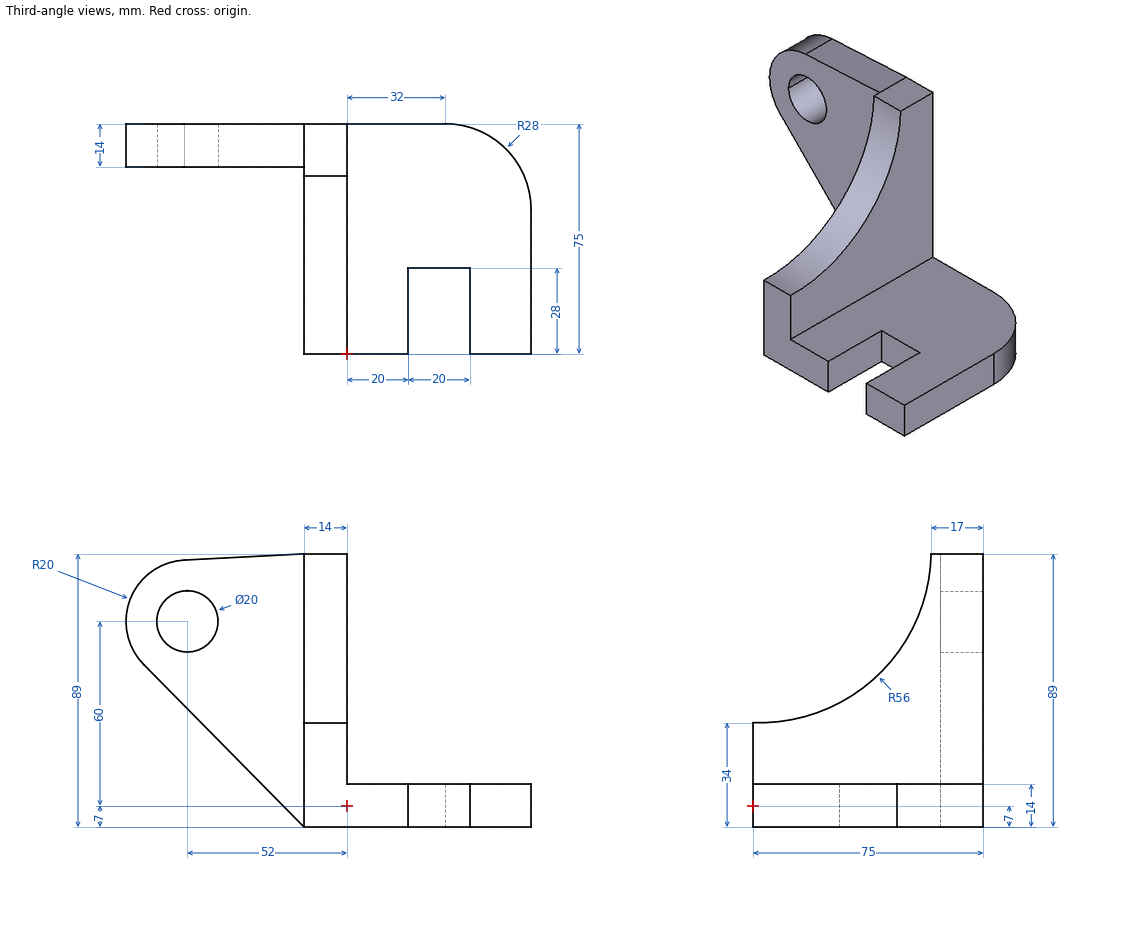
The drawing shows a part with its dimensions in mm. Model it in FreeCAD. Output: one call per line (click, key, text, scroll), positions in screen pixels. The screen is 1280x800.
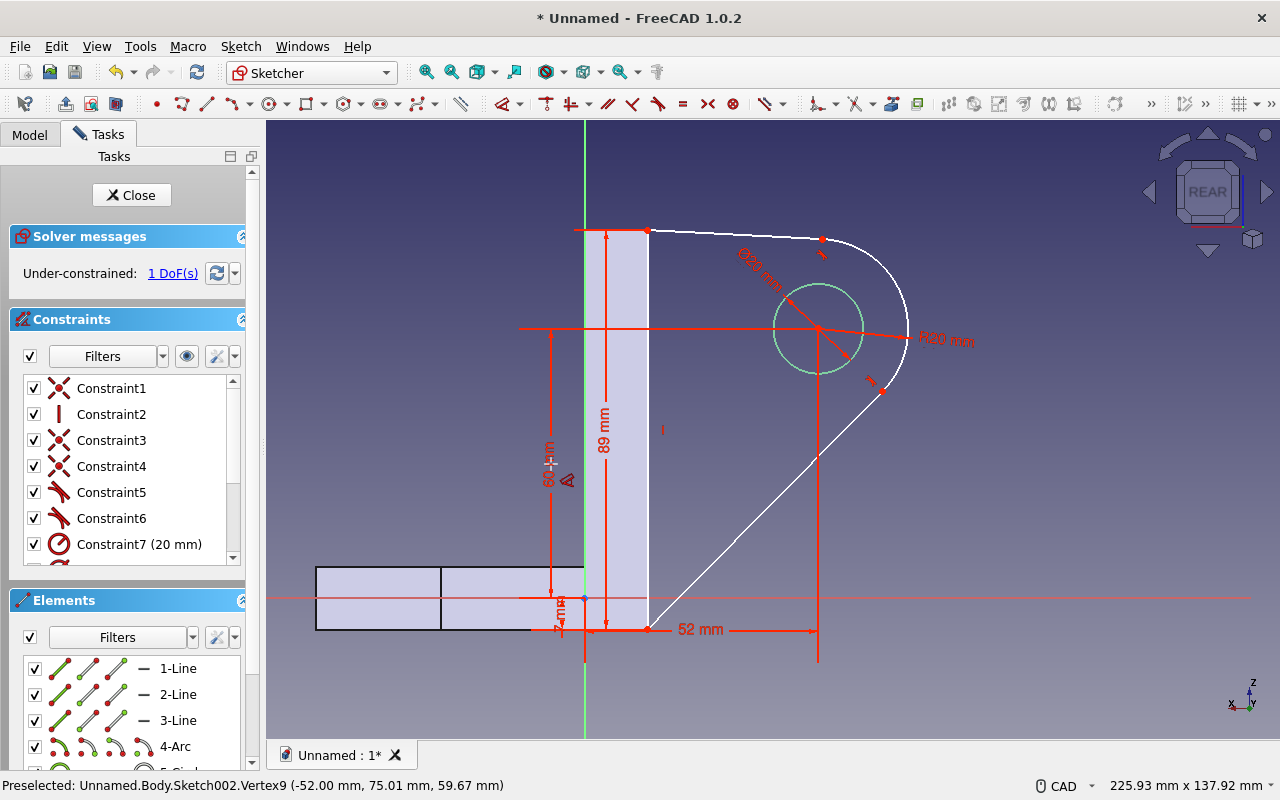
click(648, 230)
click(616, 196)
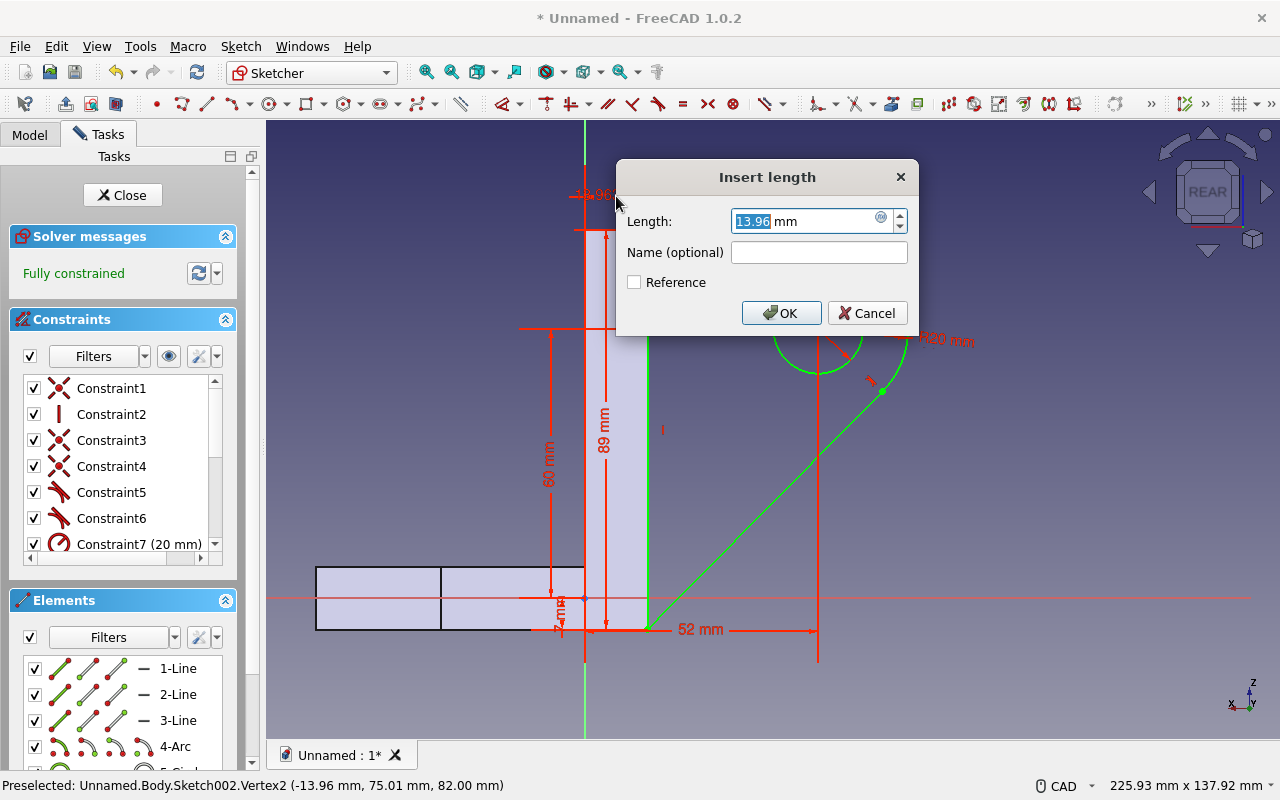
text(14)
key(Return)
key(Escape)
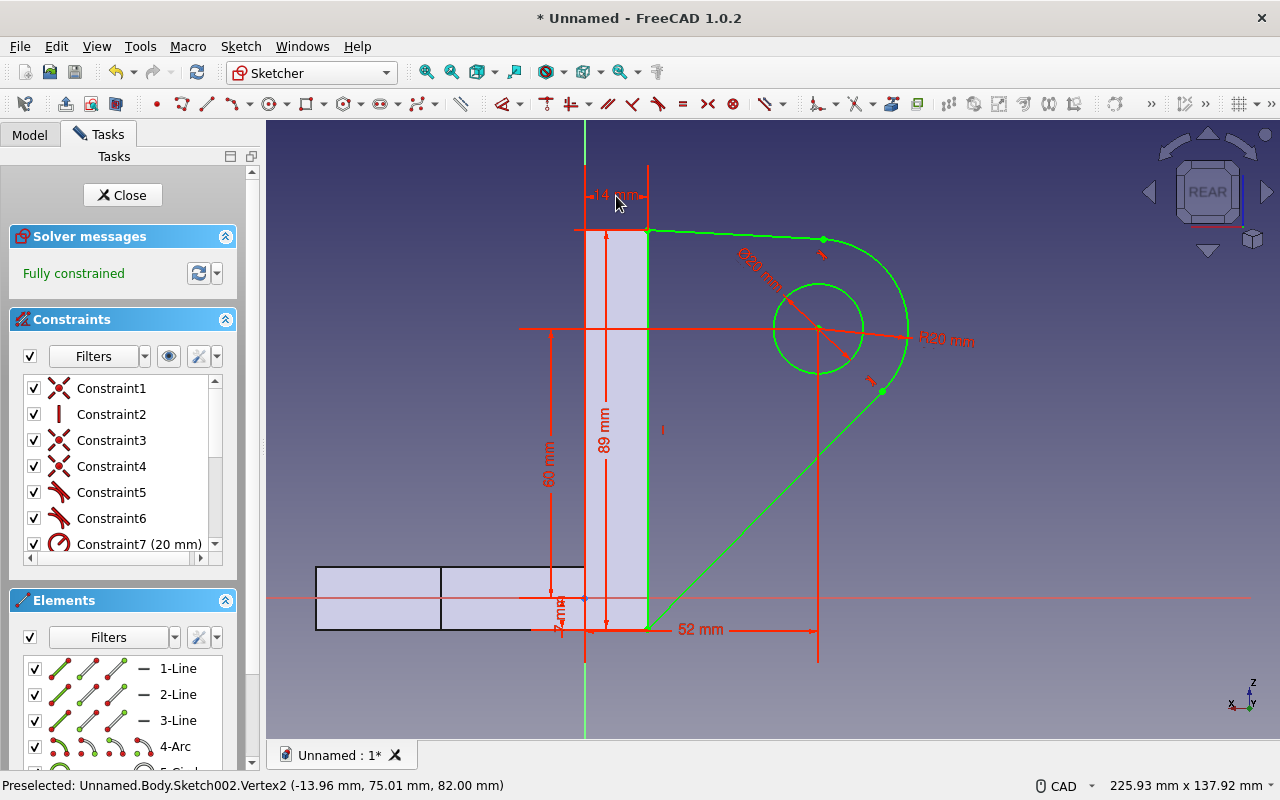
click(123, 195)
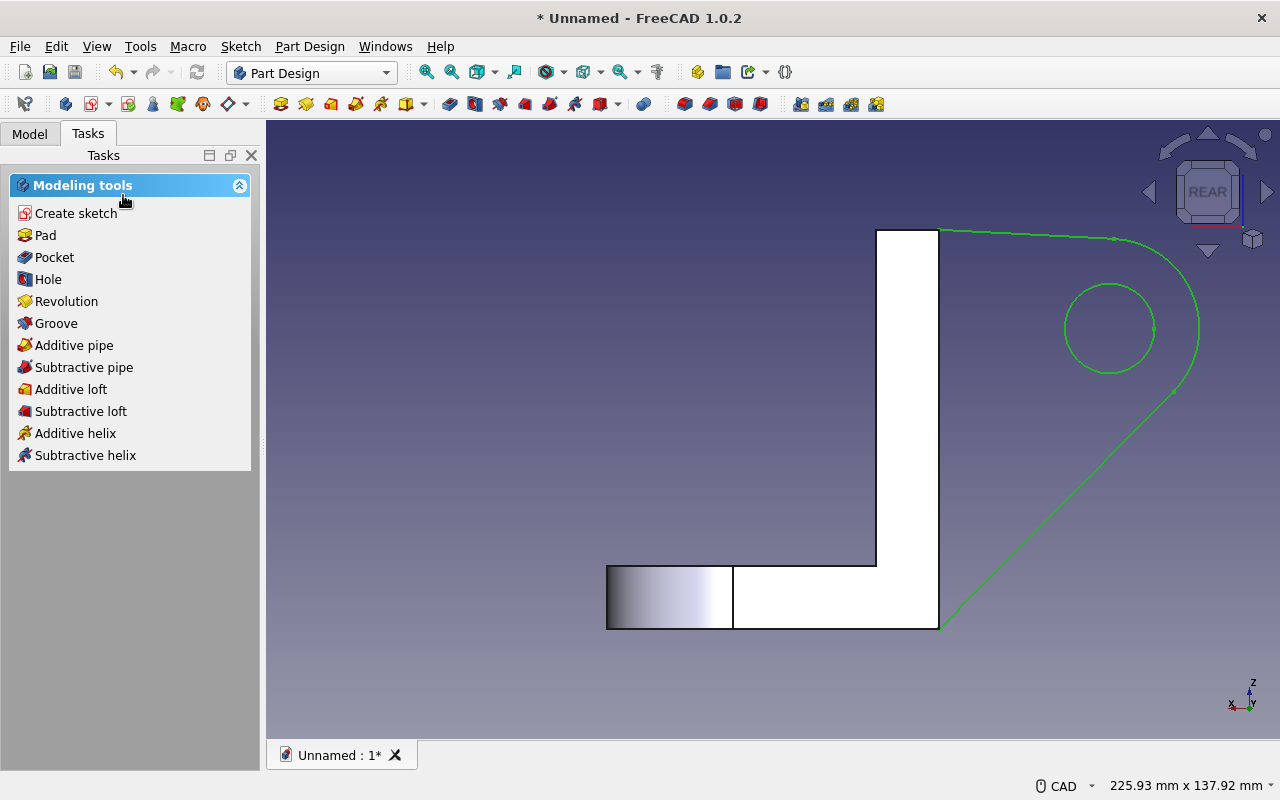
click(281, 104)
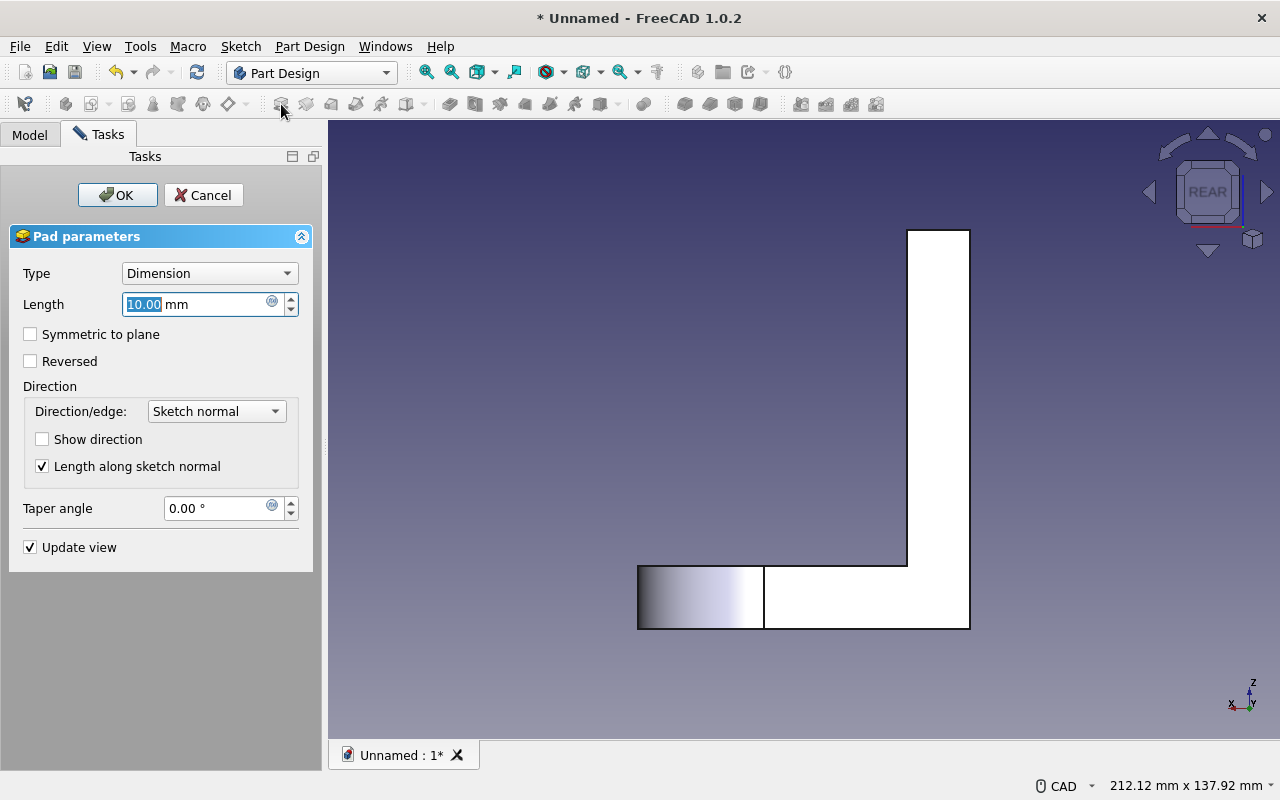
text(14)
key(Tab)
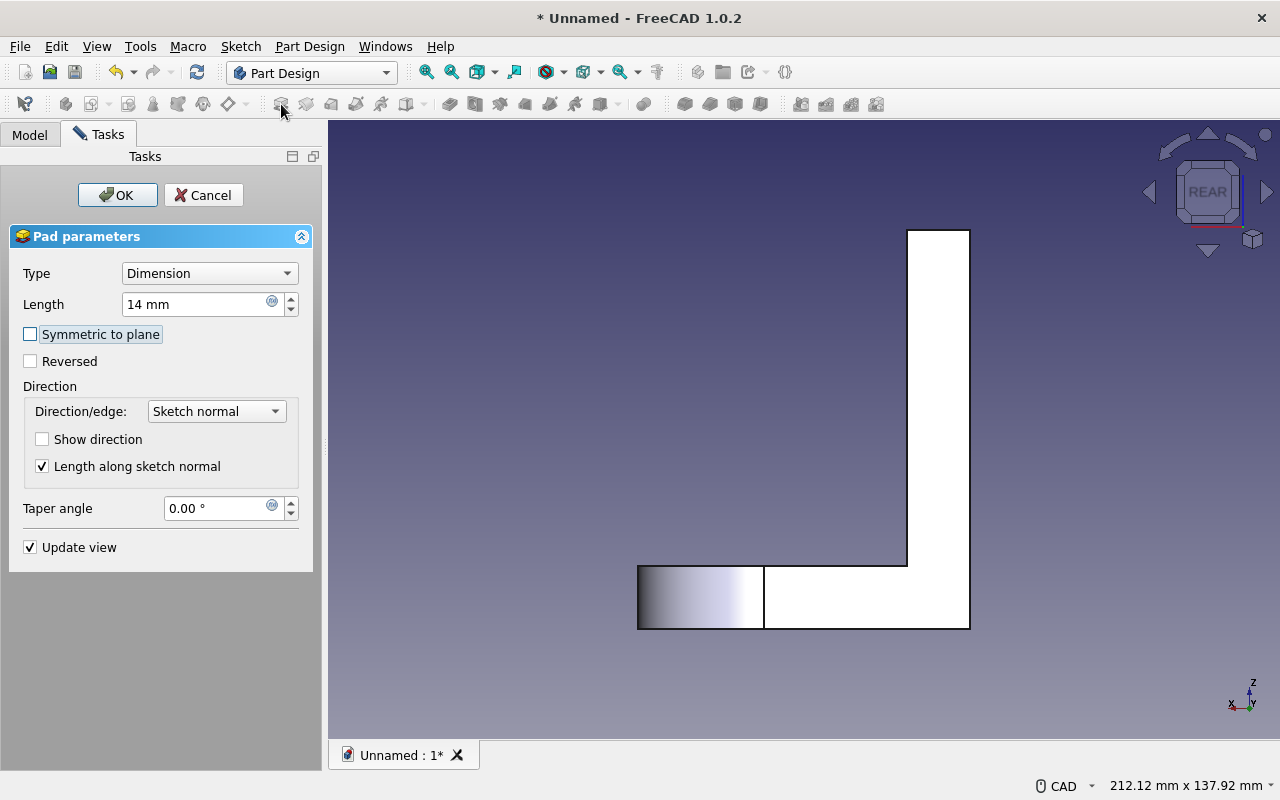
click(31, 361)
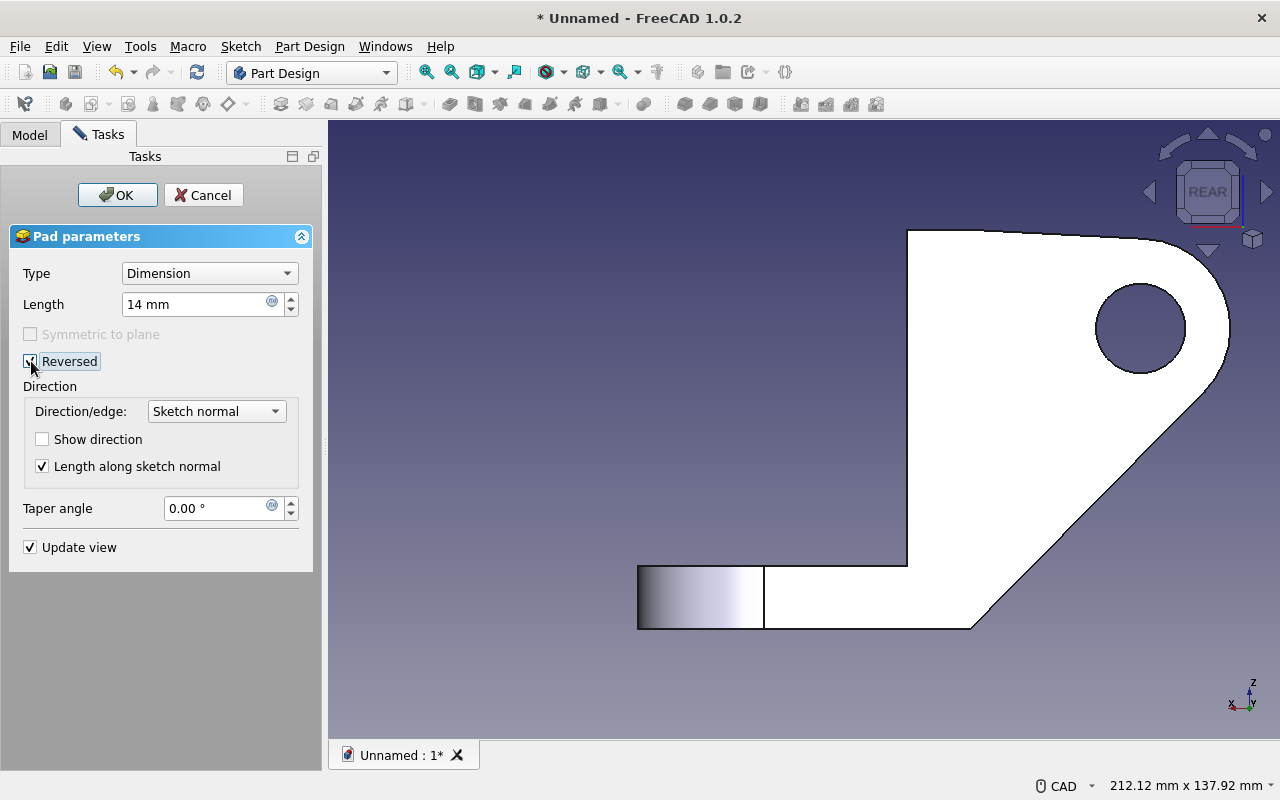
click(118, 195)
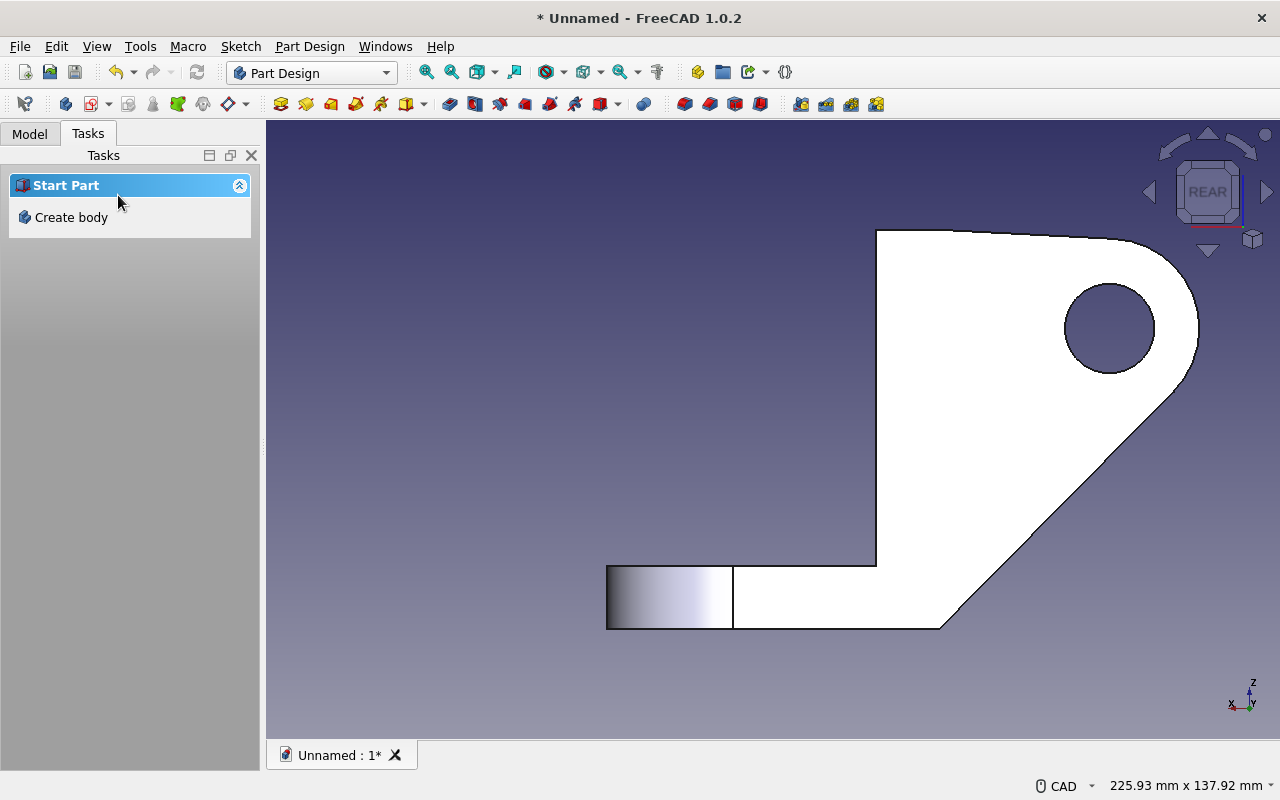
key(0)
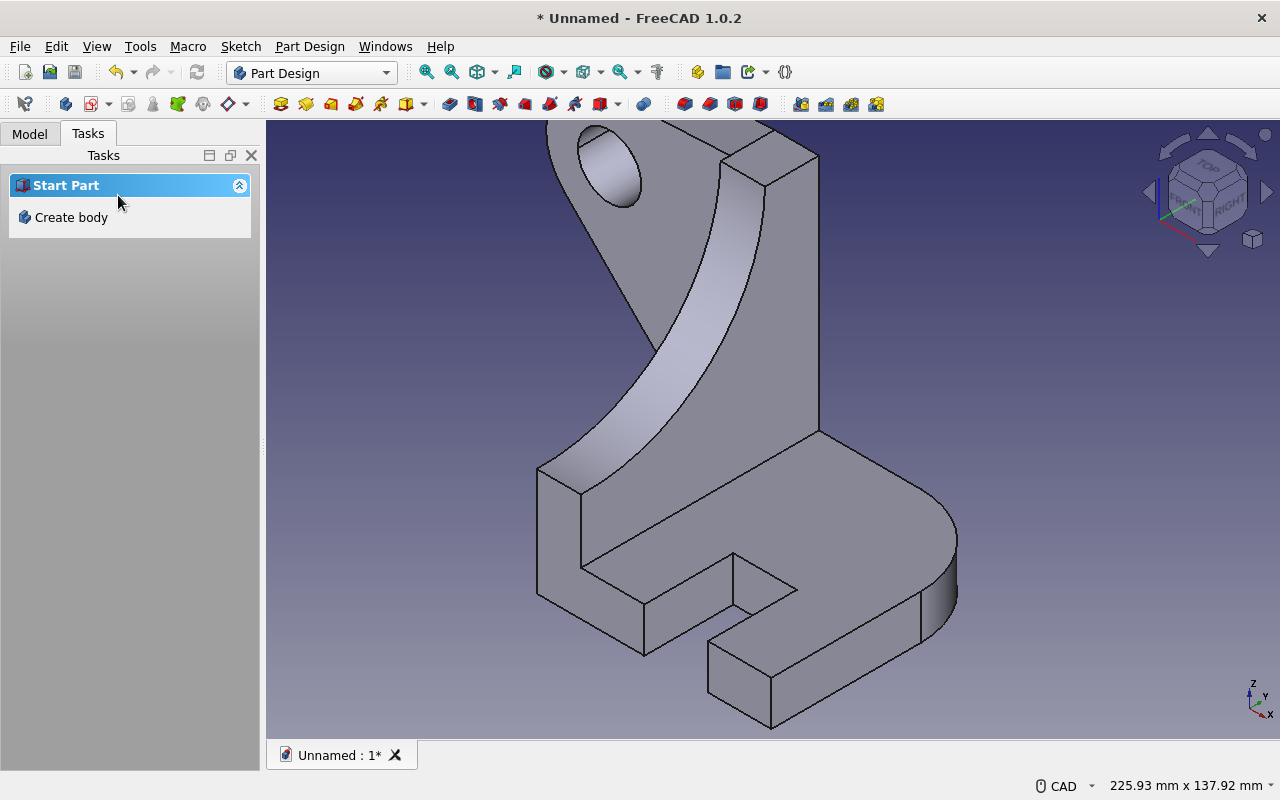
click(427, 72)